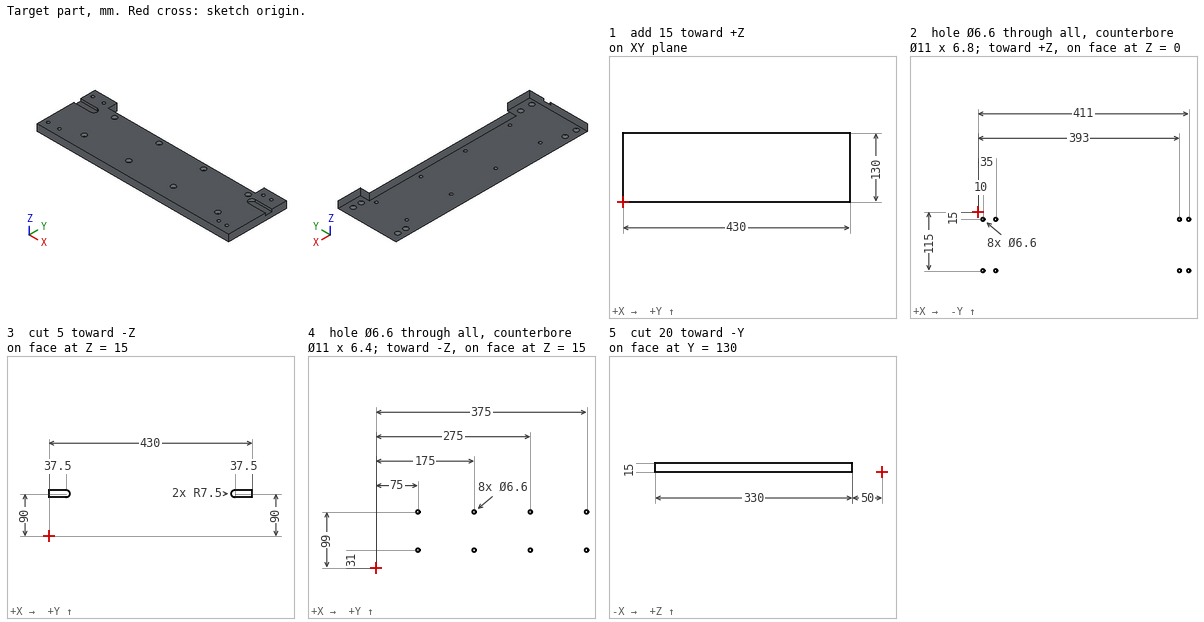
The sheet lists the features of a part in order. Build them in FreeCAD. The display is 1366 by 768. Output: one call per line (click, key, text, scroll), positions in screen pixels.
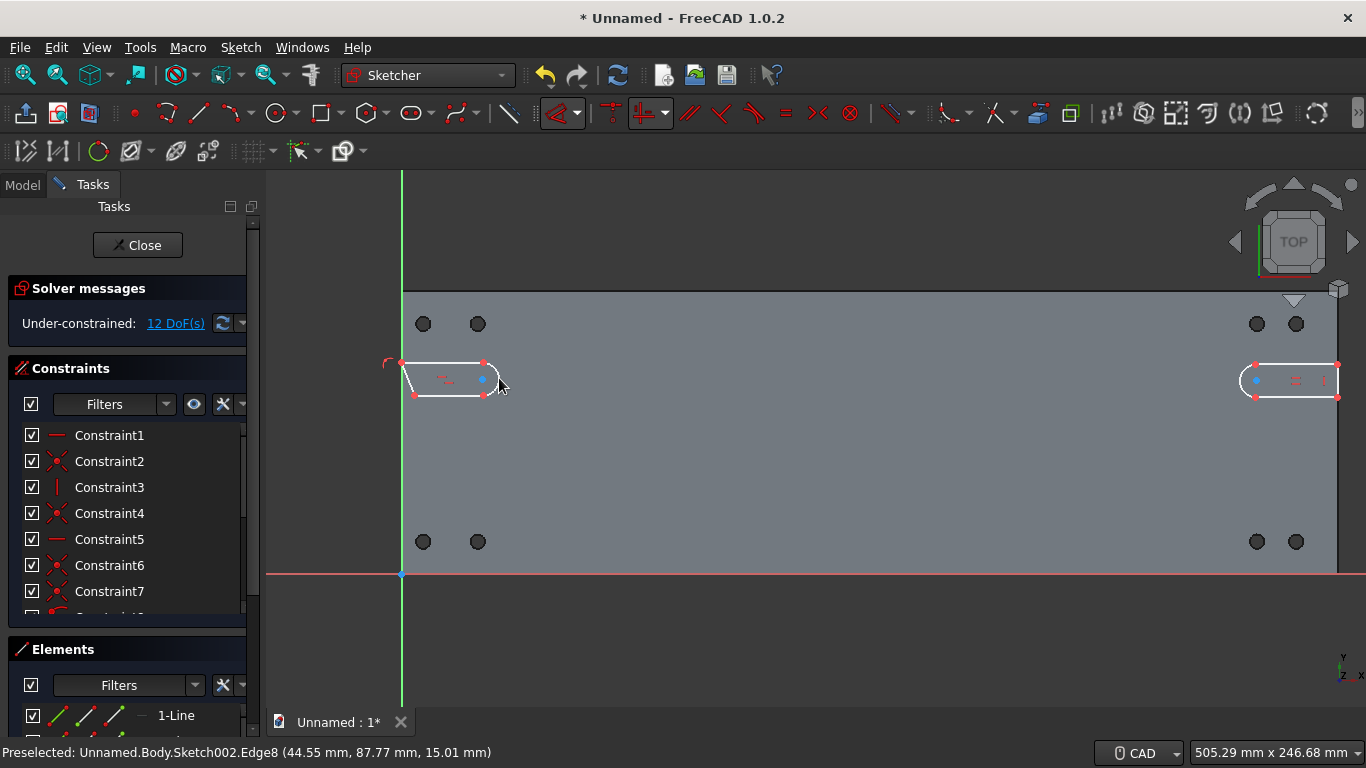
scroll(499, 378, down, 2)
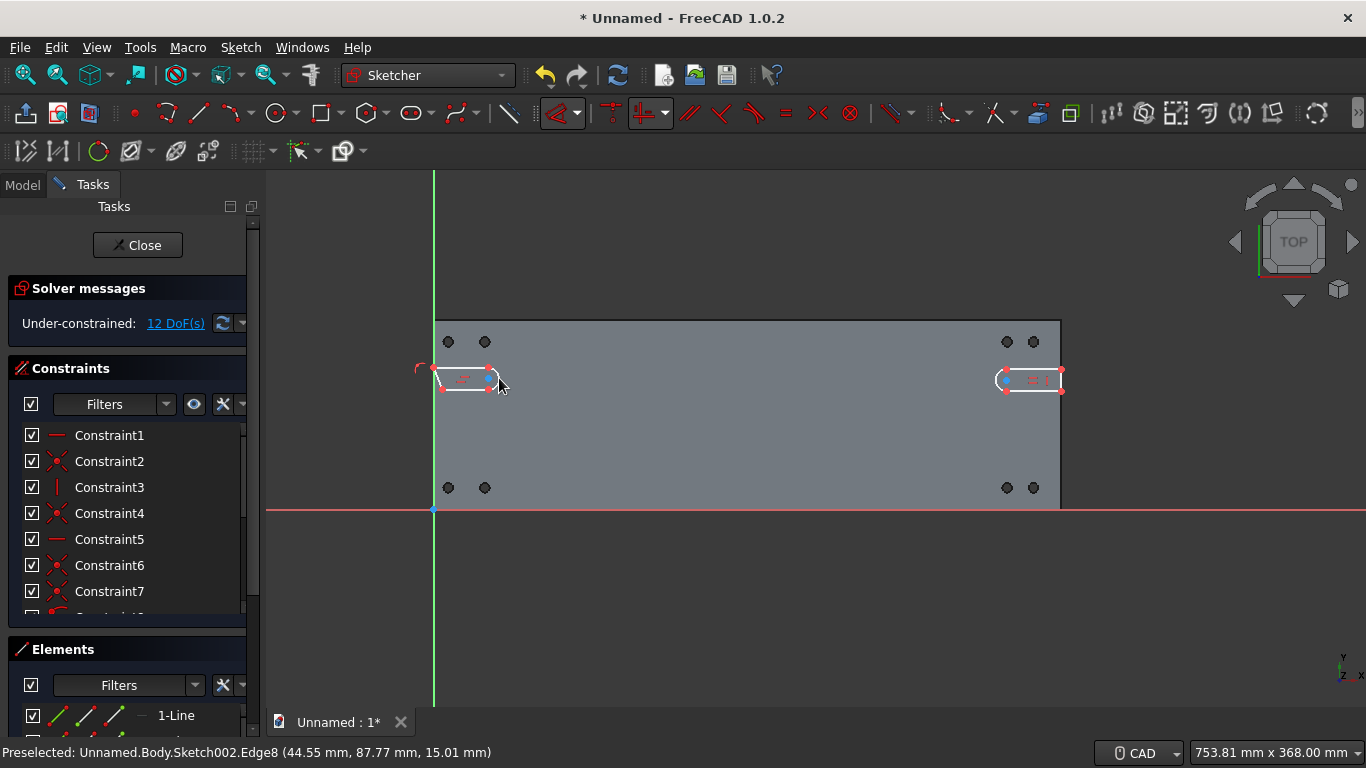
click(1023, 391)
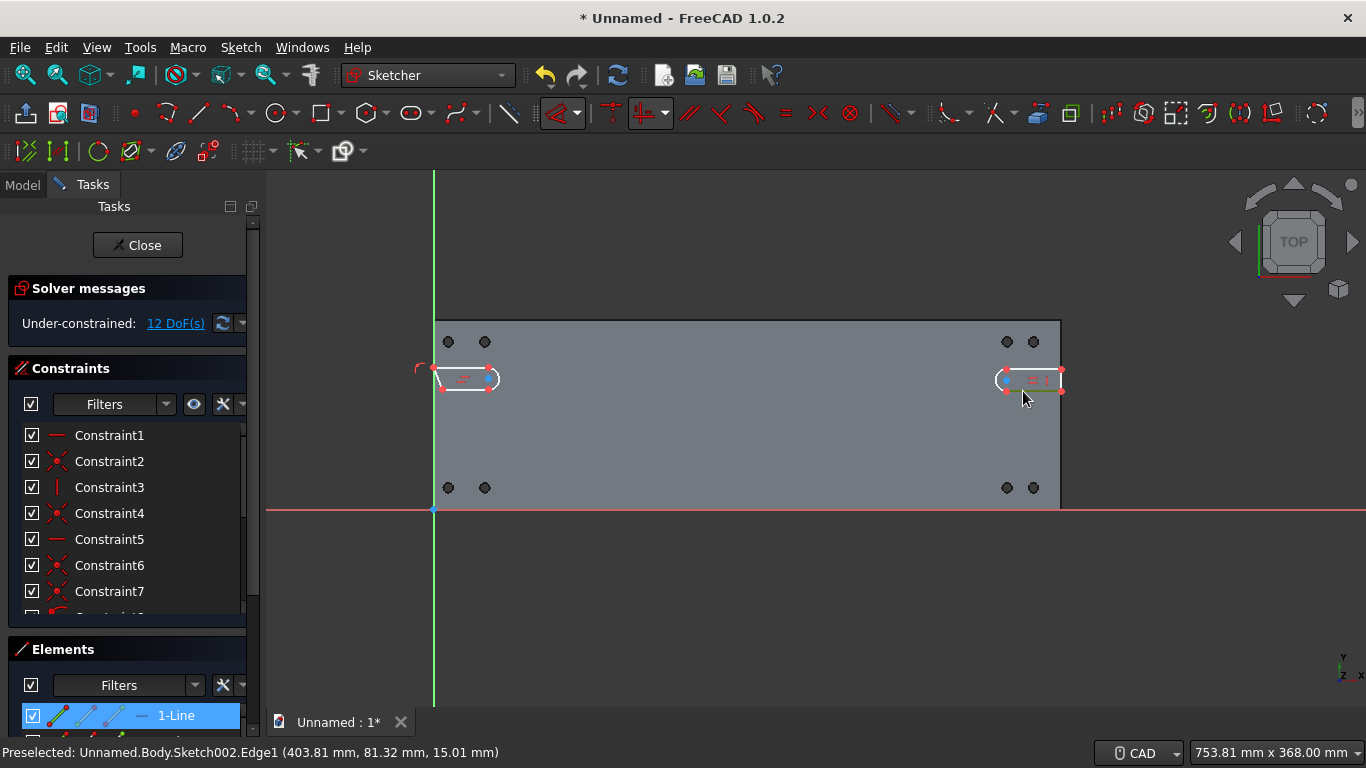
scroll(998, 374, up, 2)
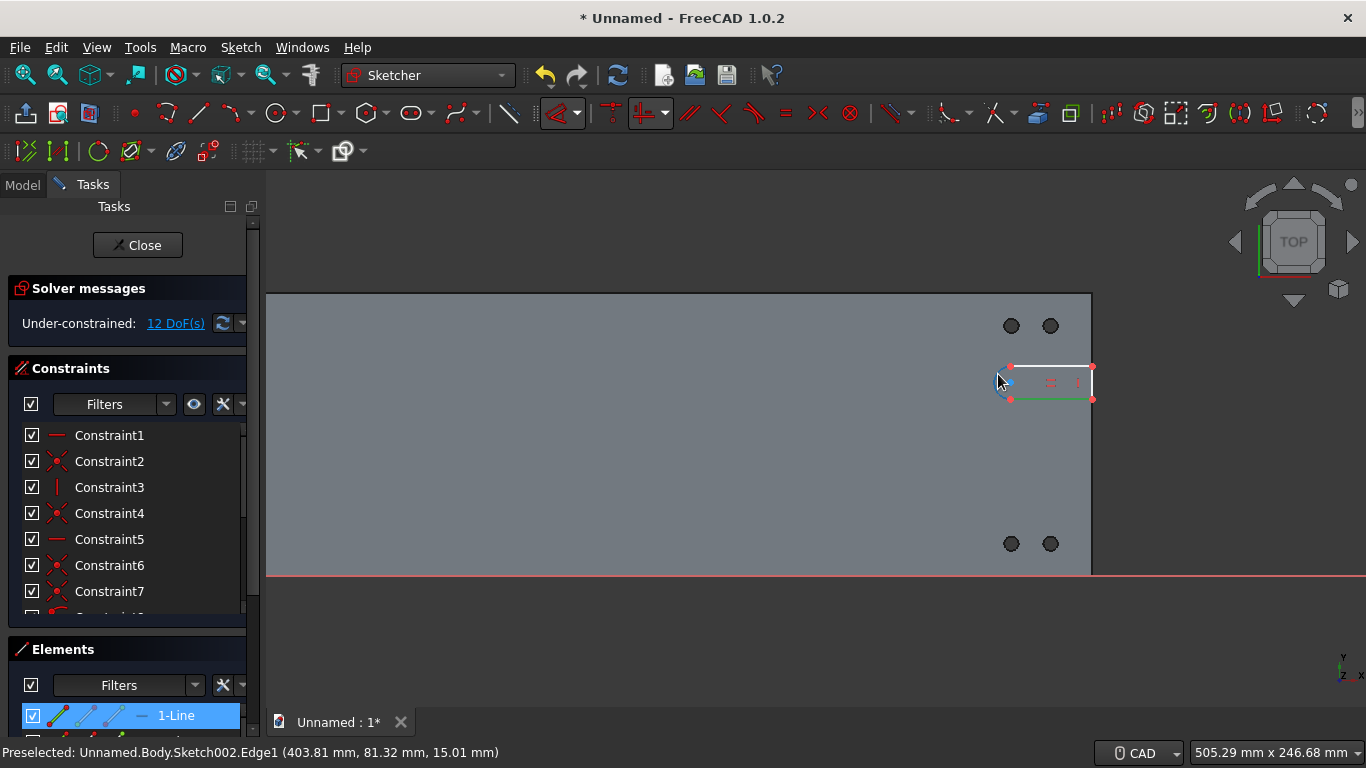
click(997, 373)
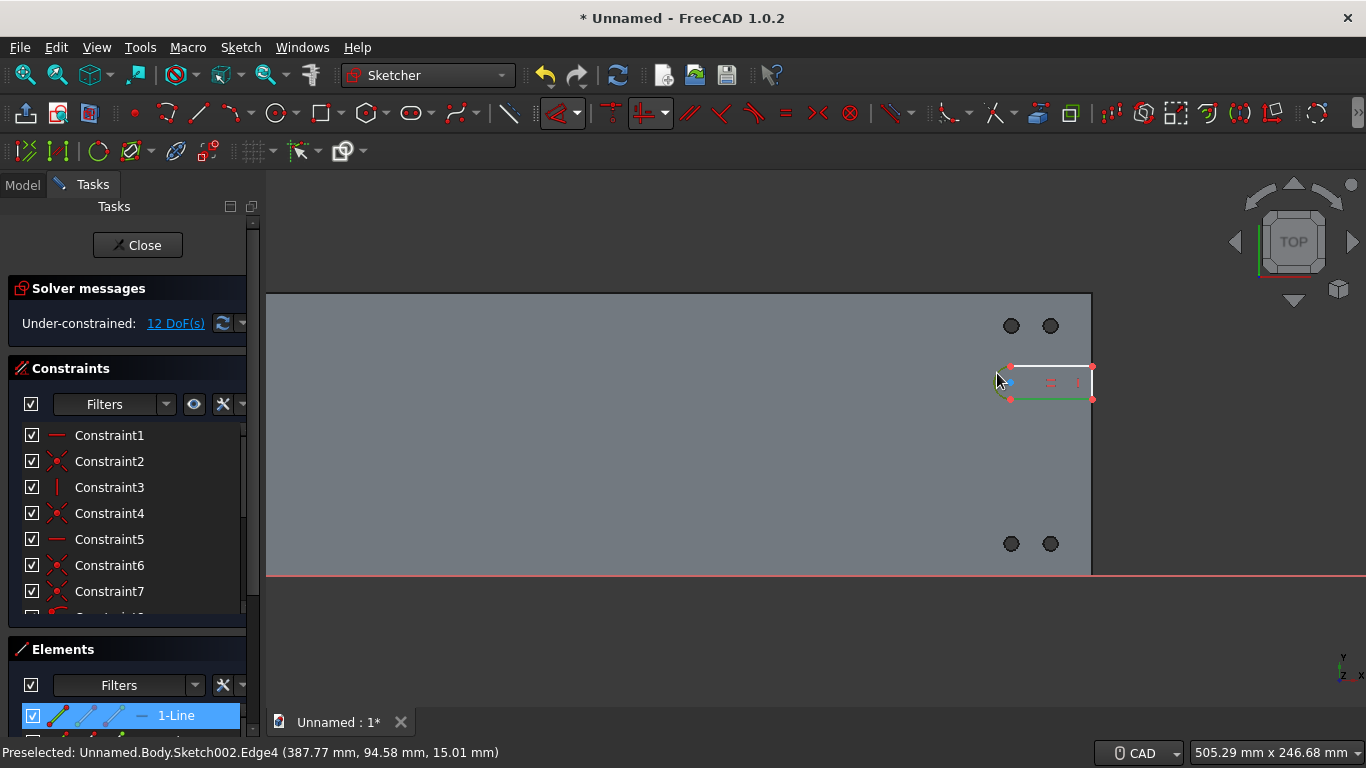
click(754, 114)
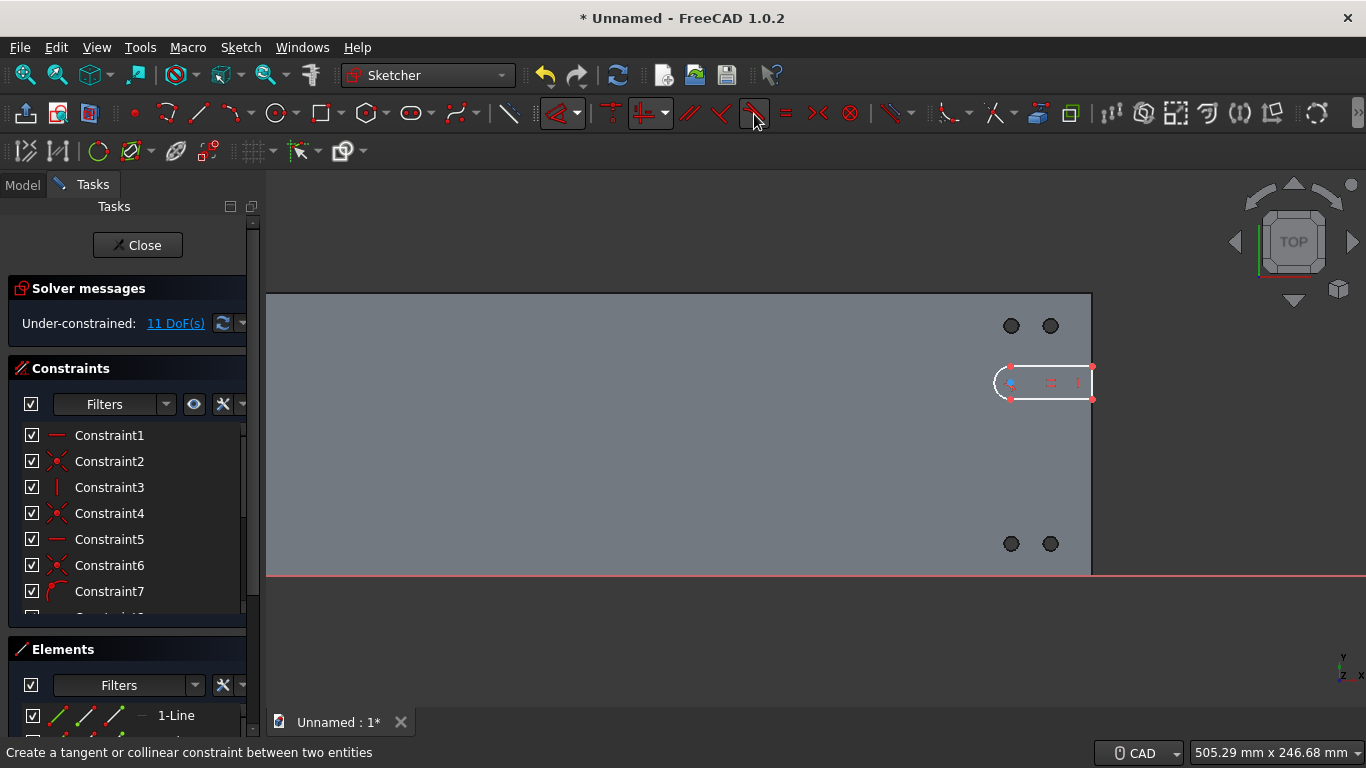
click(1068, 366)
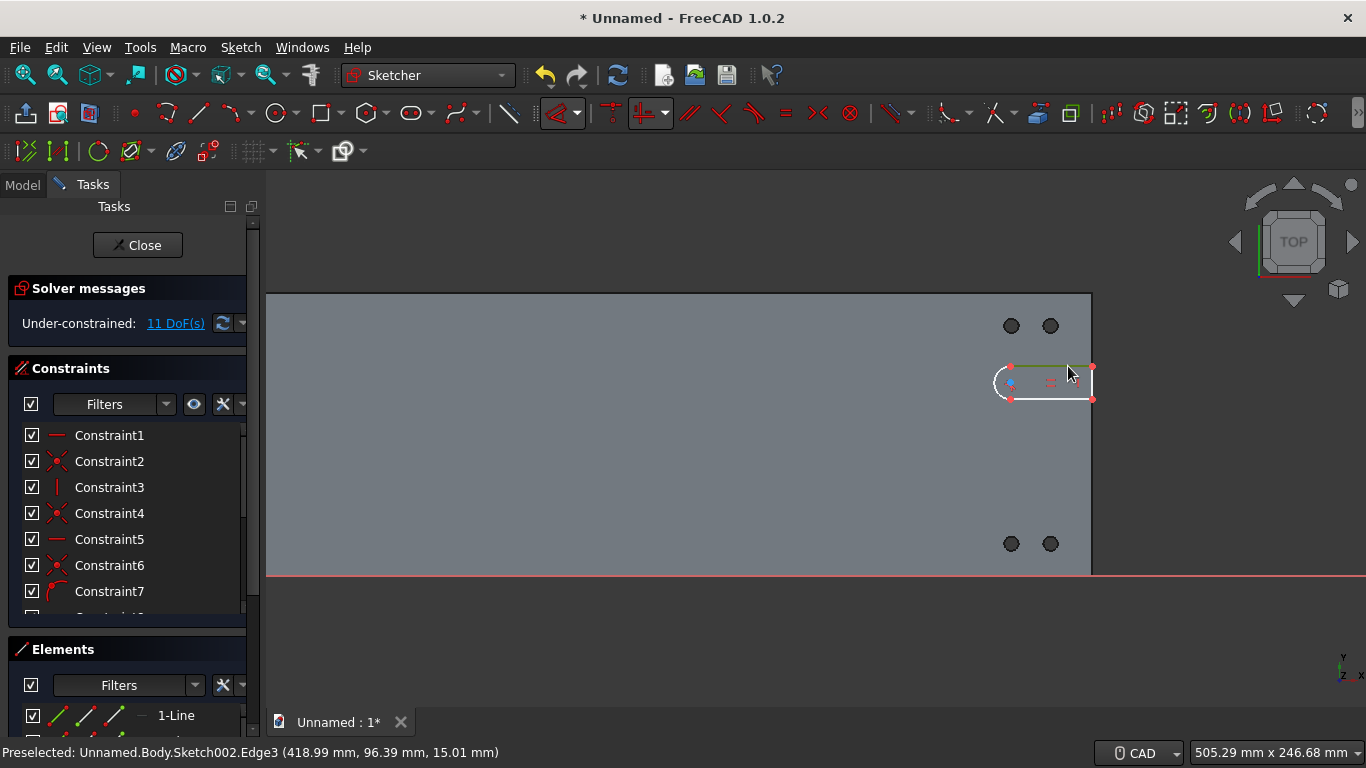
click(997, 374)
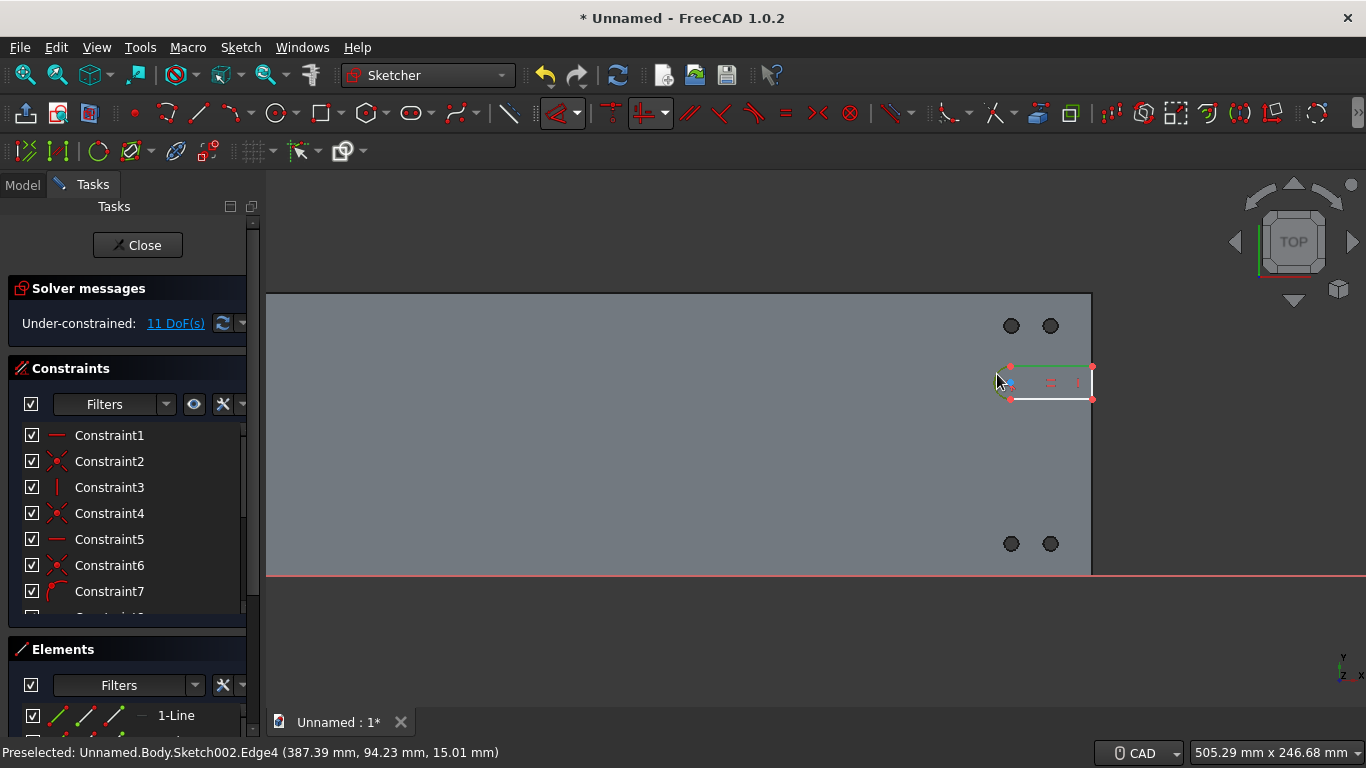
click(754, 114)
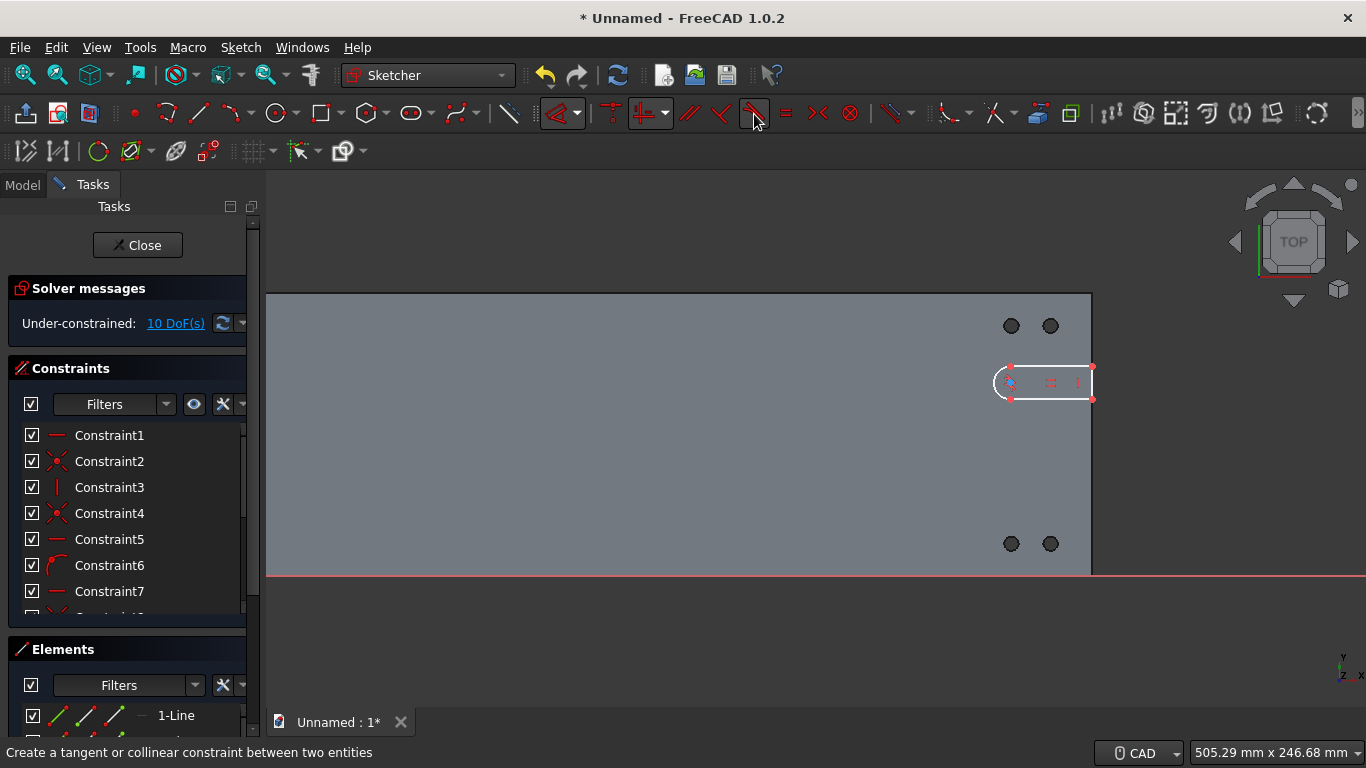
scroll(999, 374, down, 2)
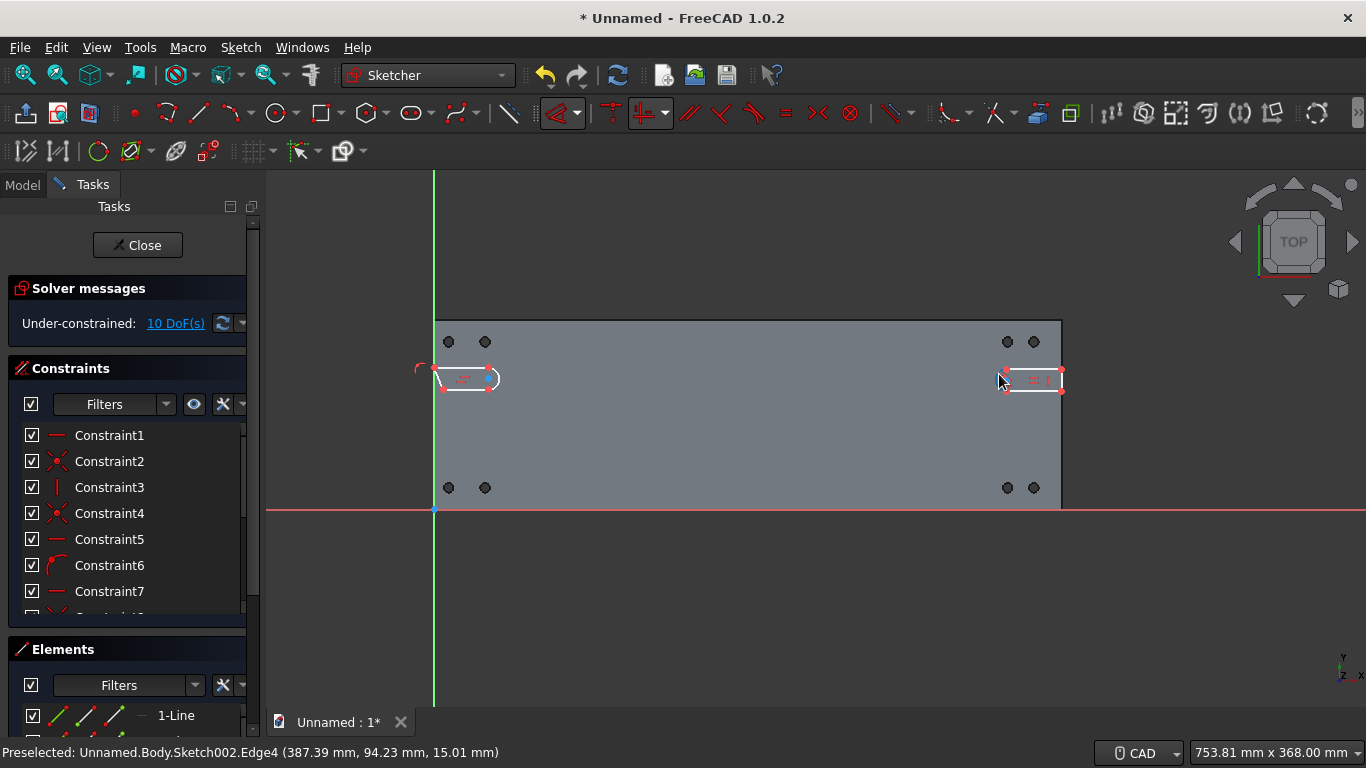
click(473, 368)